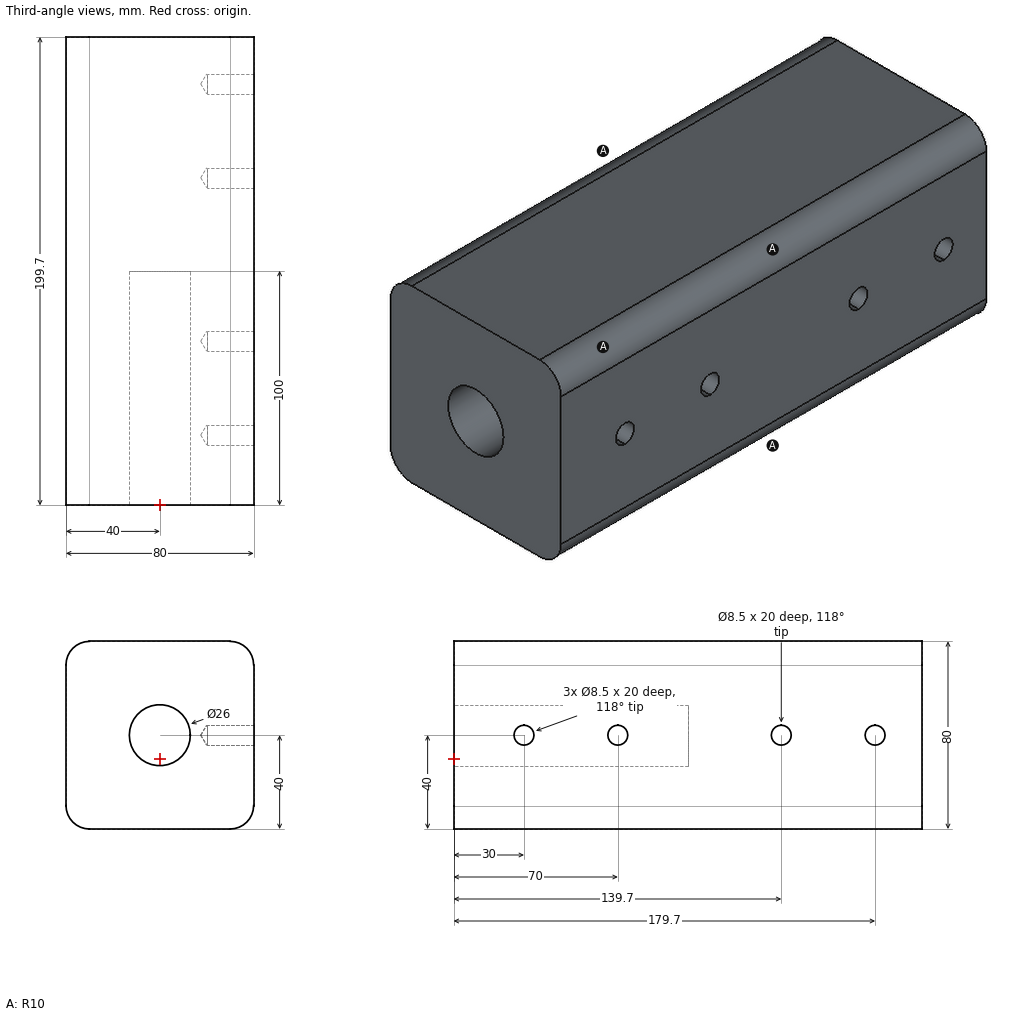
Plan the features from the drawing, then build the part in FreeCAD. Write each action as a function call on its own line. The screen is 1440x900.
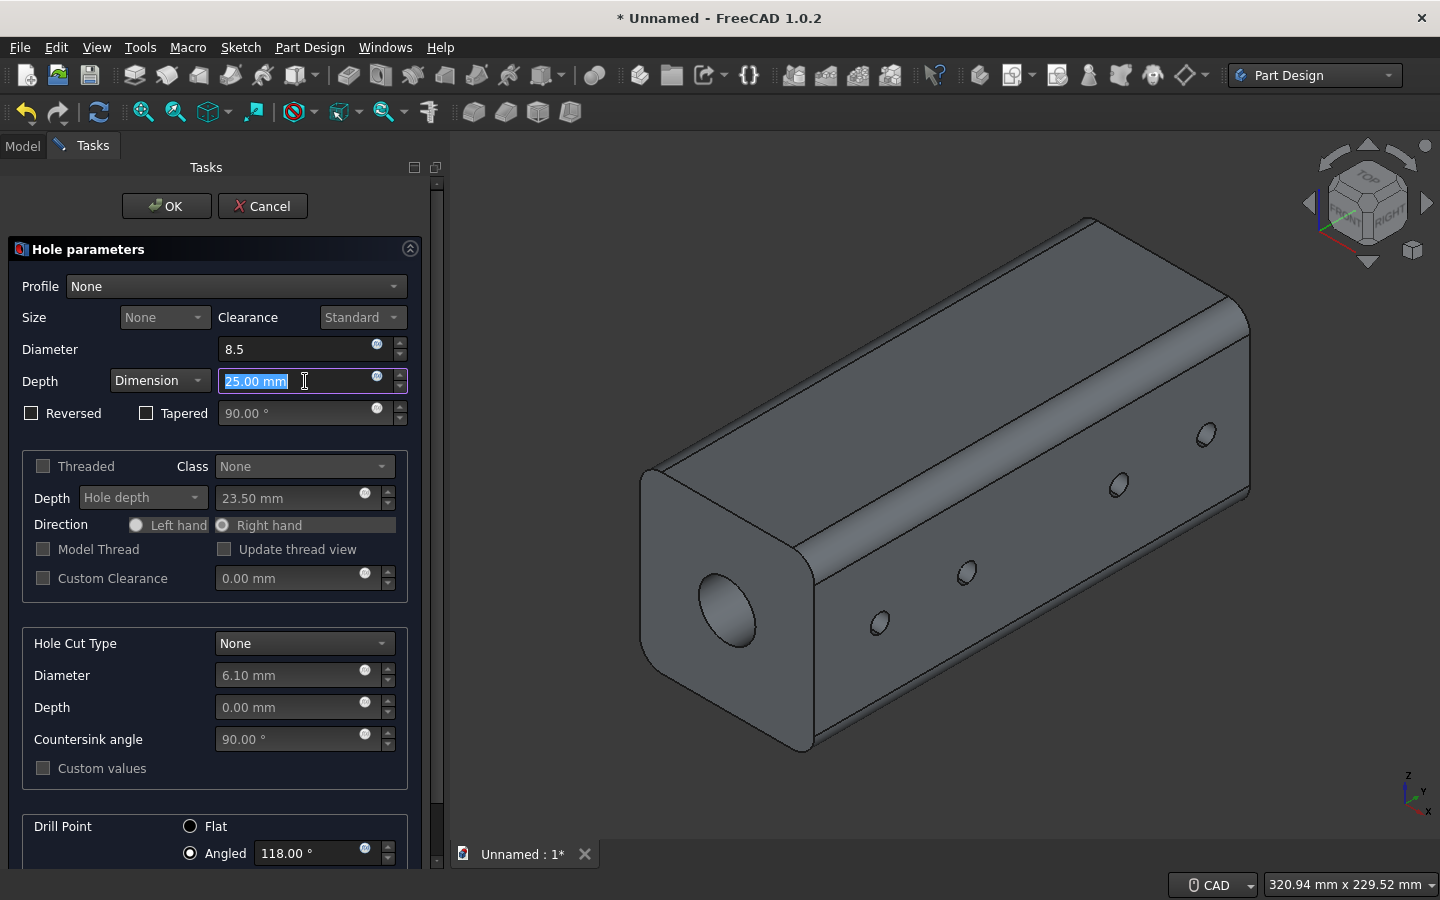
text(20)
key(Tab)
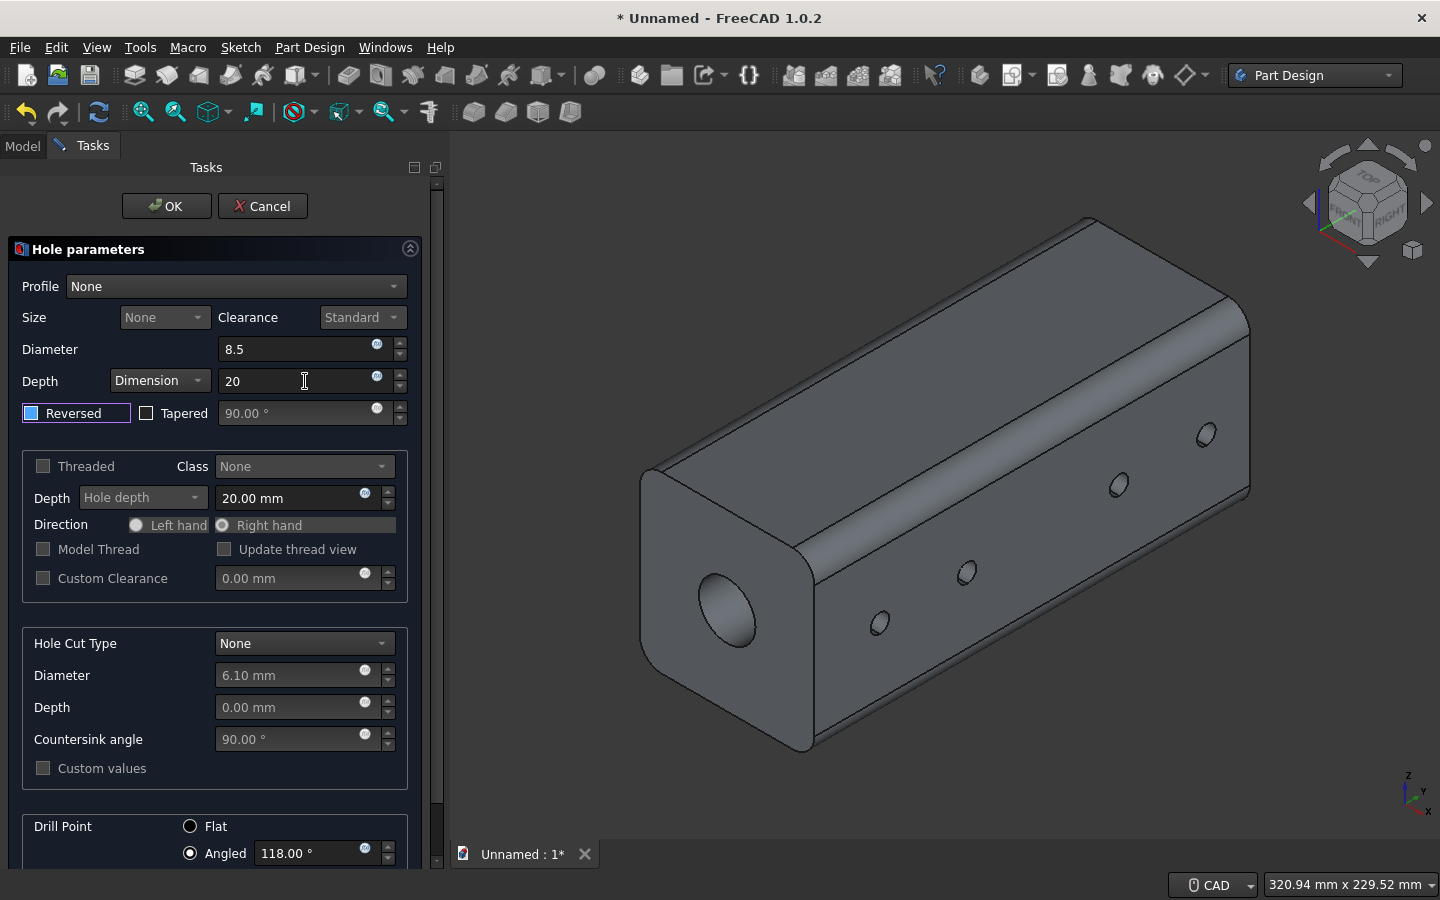
click(167, 206)